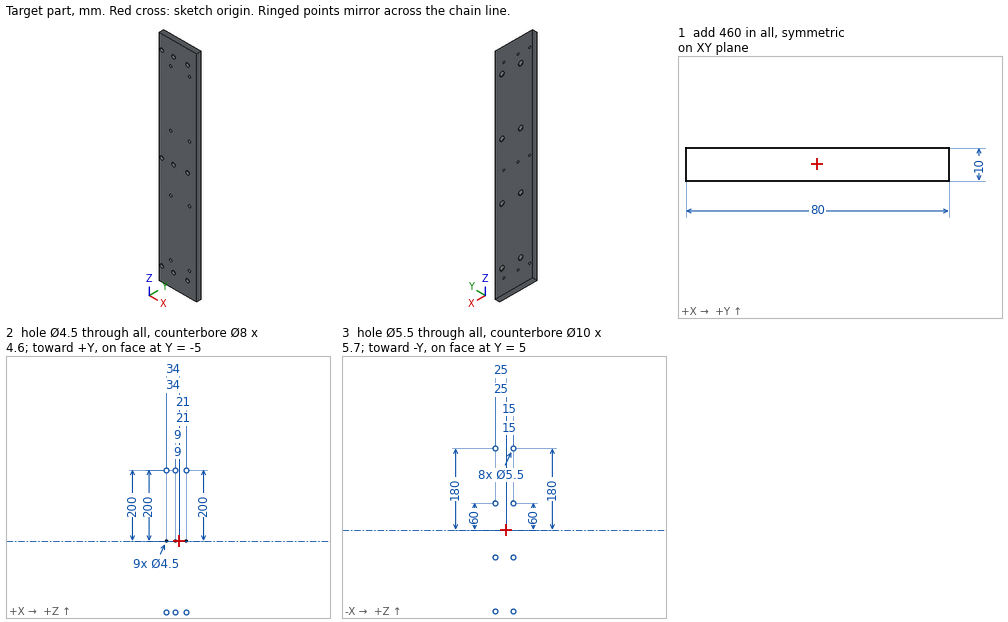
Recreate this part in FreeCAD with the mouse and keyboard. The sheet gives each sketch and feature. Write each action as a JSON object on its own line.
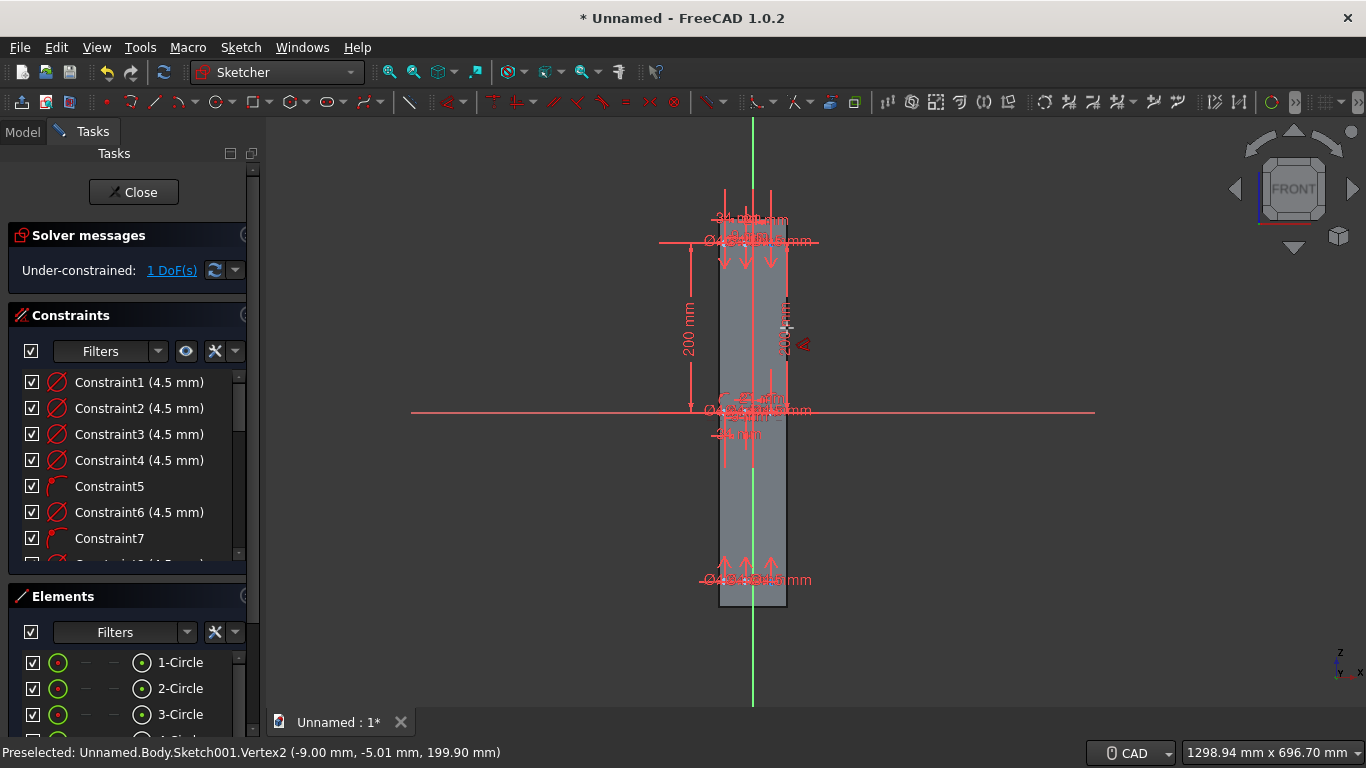
{"action": "left_click", "coordinate": [771, 243]}
{"action": "left_click", "coordinate": [805, 289]}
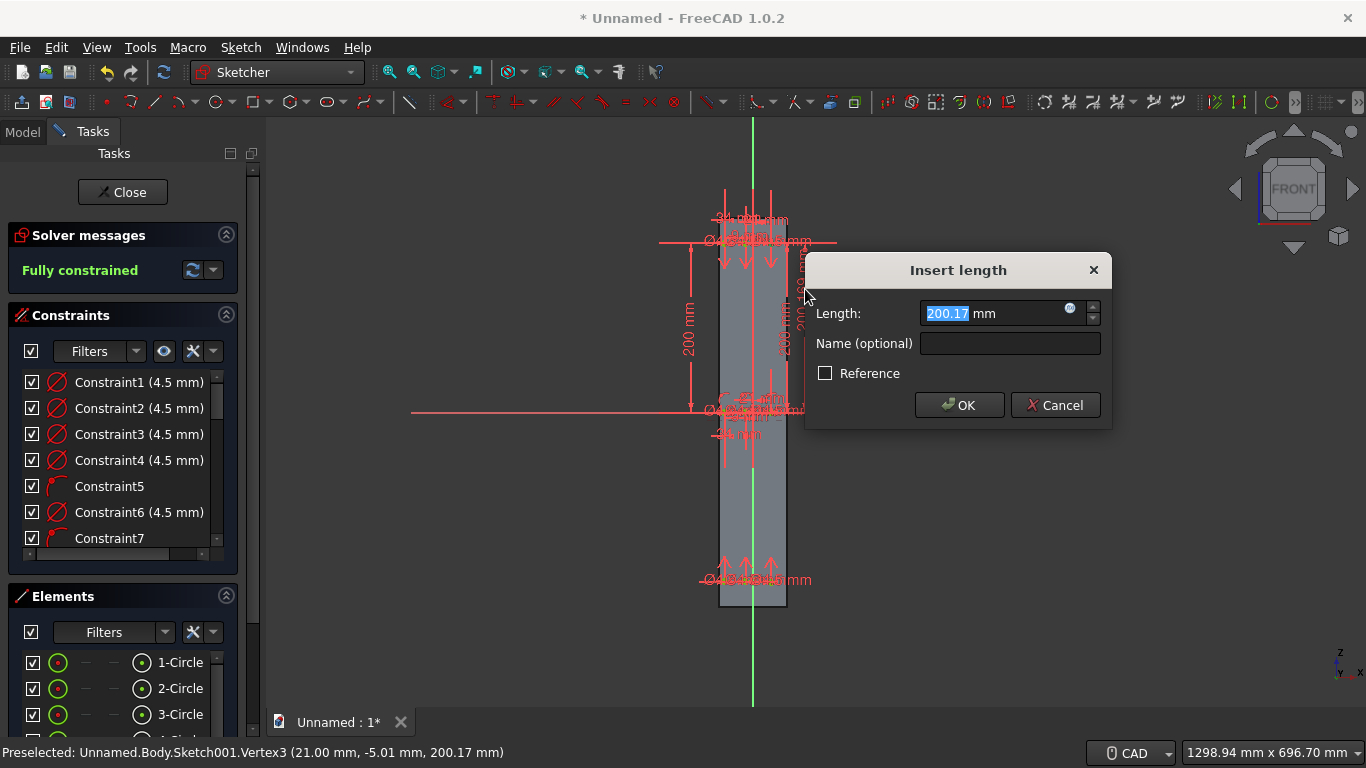
{"action": "type", "text": "200"}
{"action": "key", "text": "Return"}
{"action": "key", "text": "Escape"}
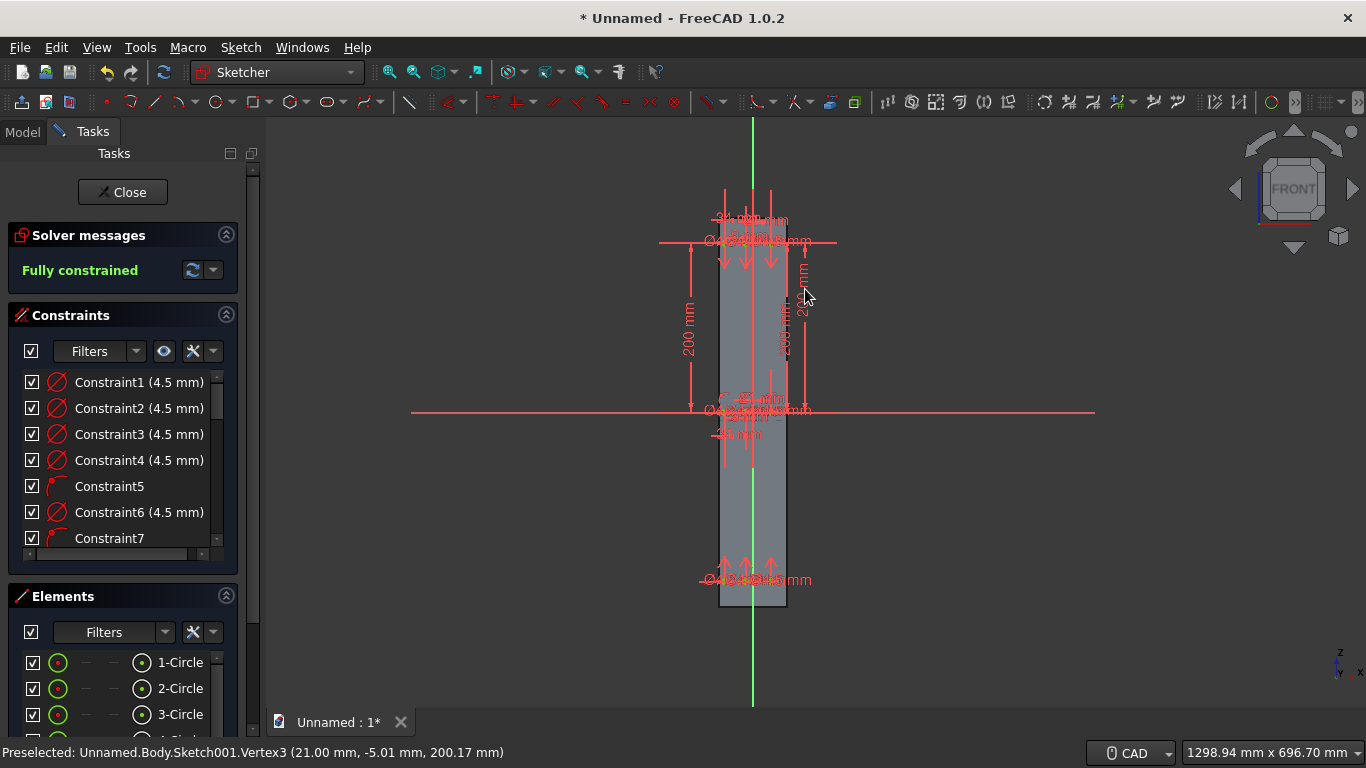
{"action": "left_click", "coordinate": [123, 192]}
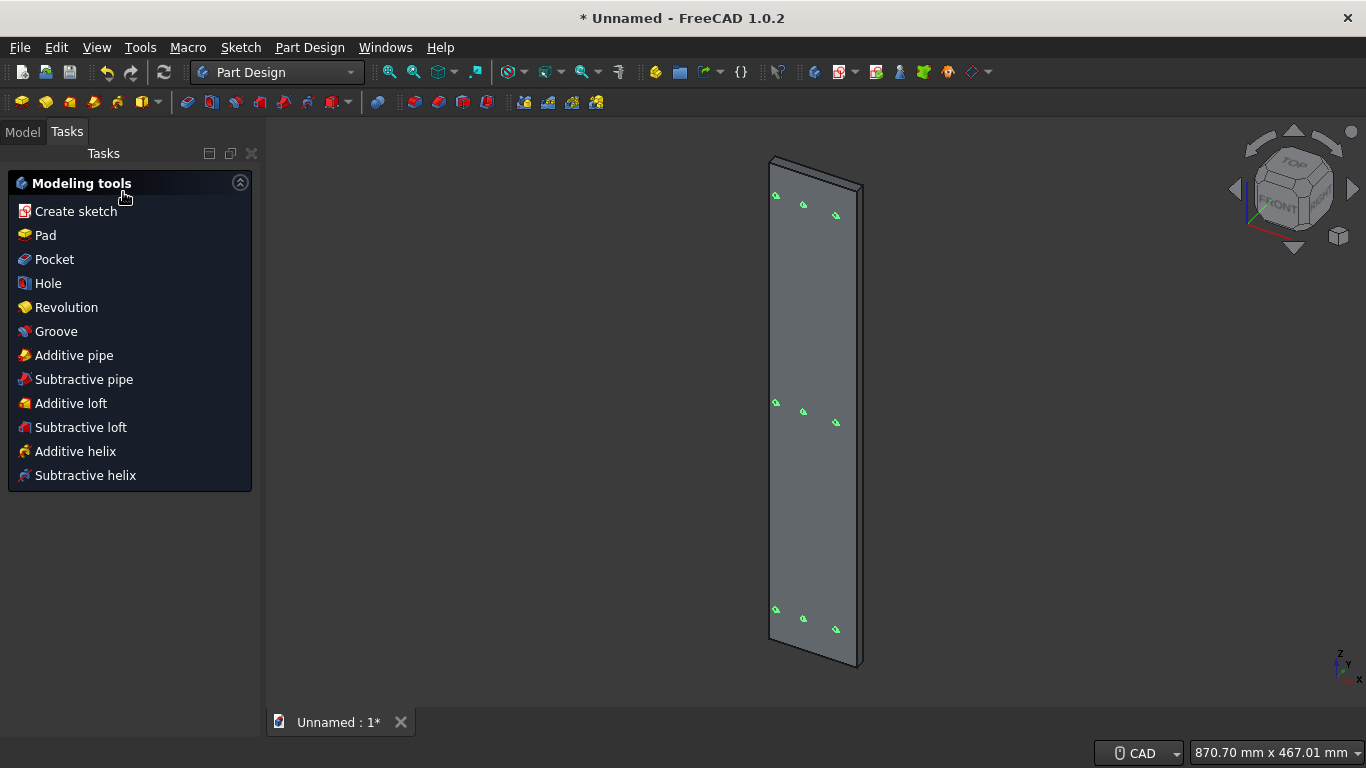
{"action": "left_click", "coordinate": [212, 102]}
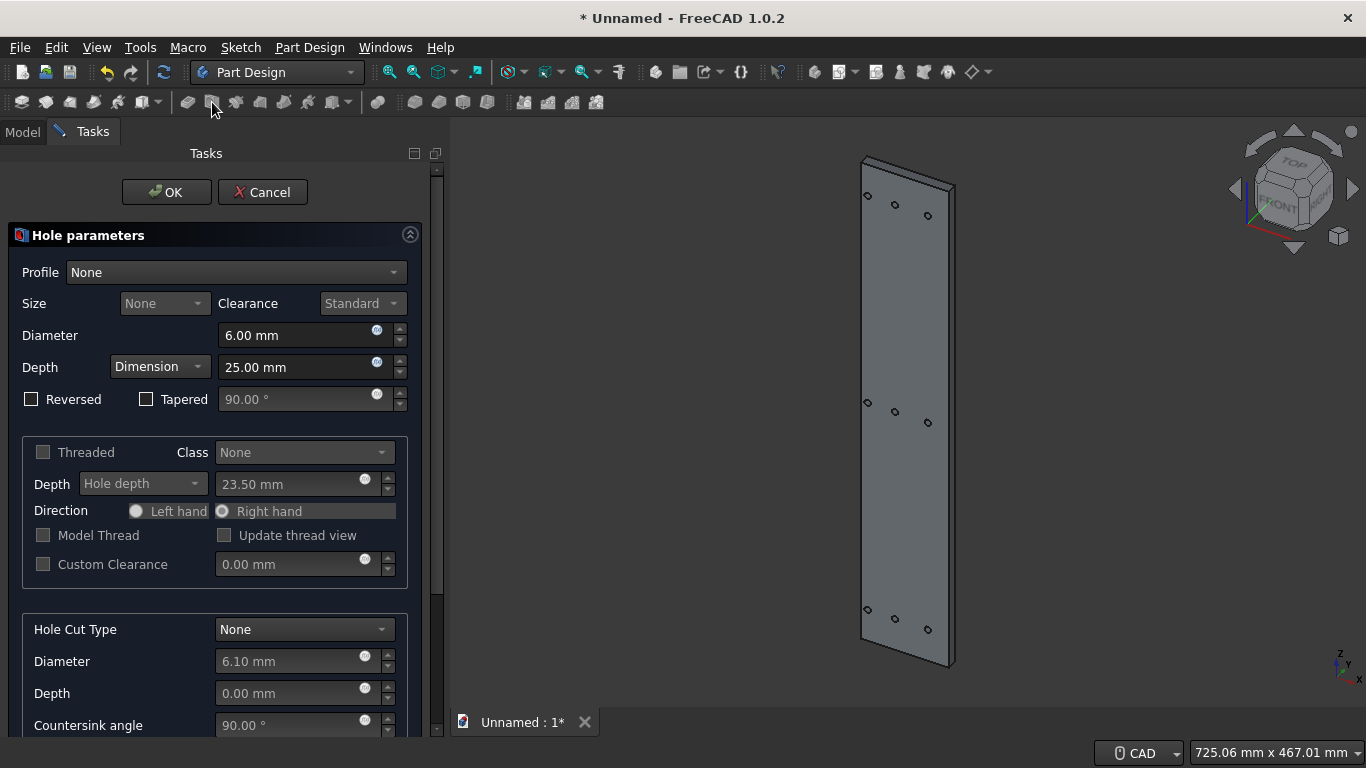
{"action": "triple_click", "coordinate": [305, 335]}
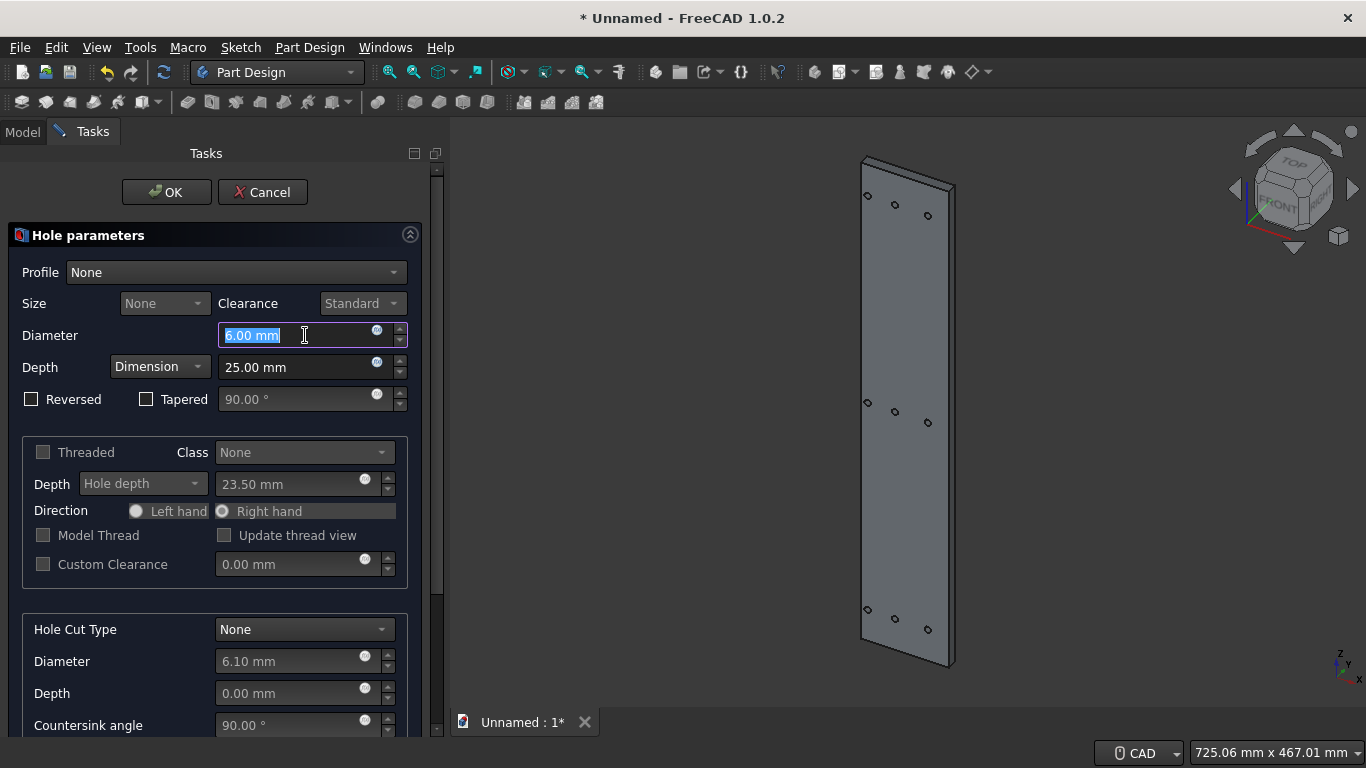
{"action": "type", "text": "4.5"}
{"action": "key", "text": "Tab"}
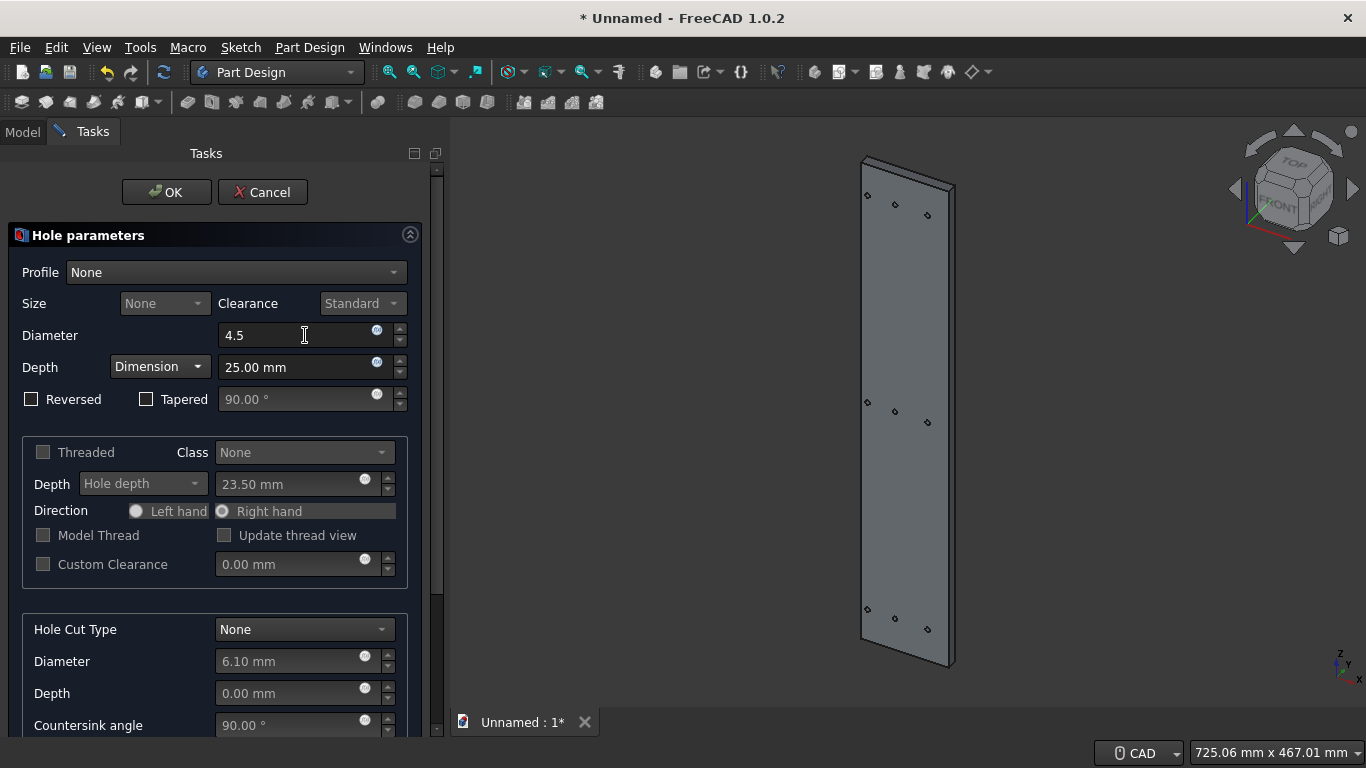
{"action": "left_click", "coordinate": [161, 366]}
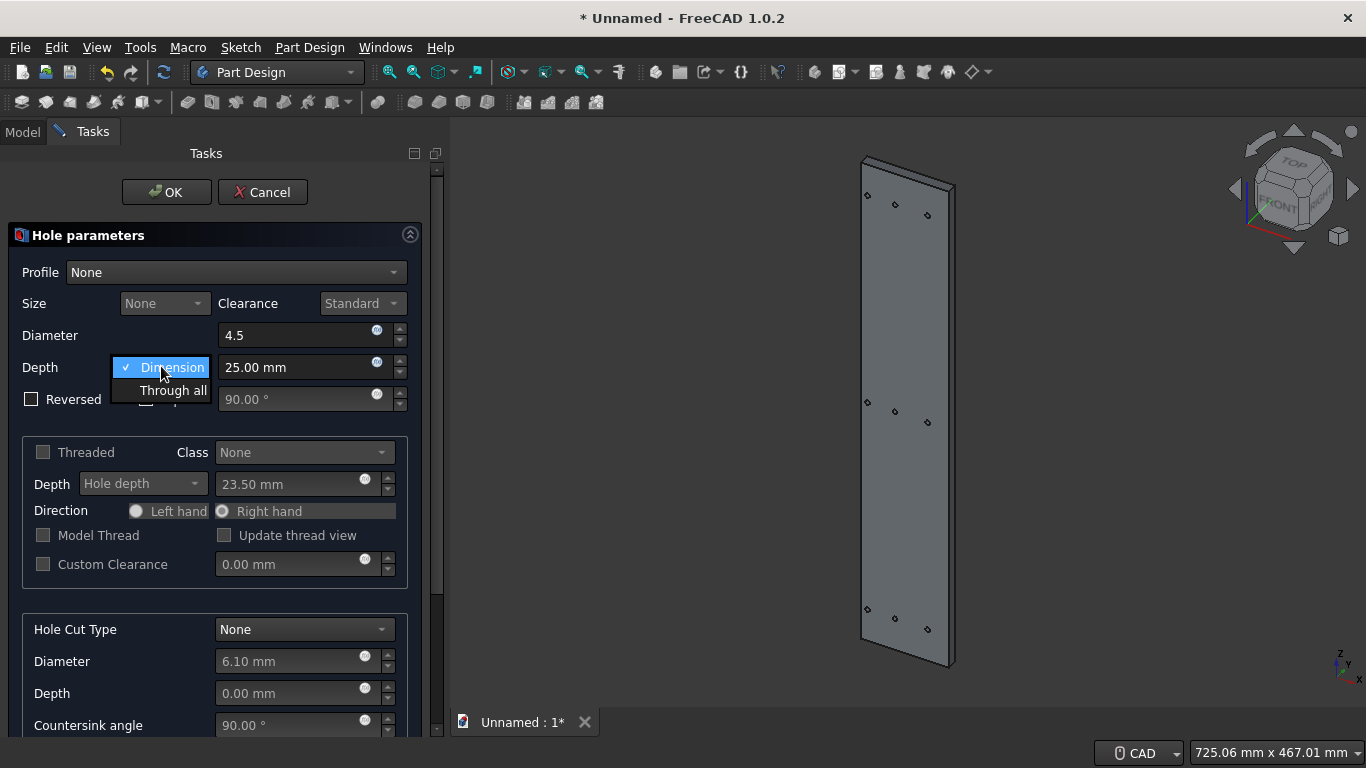
{"action": "left_click", "coordinate": [160, 390]}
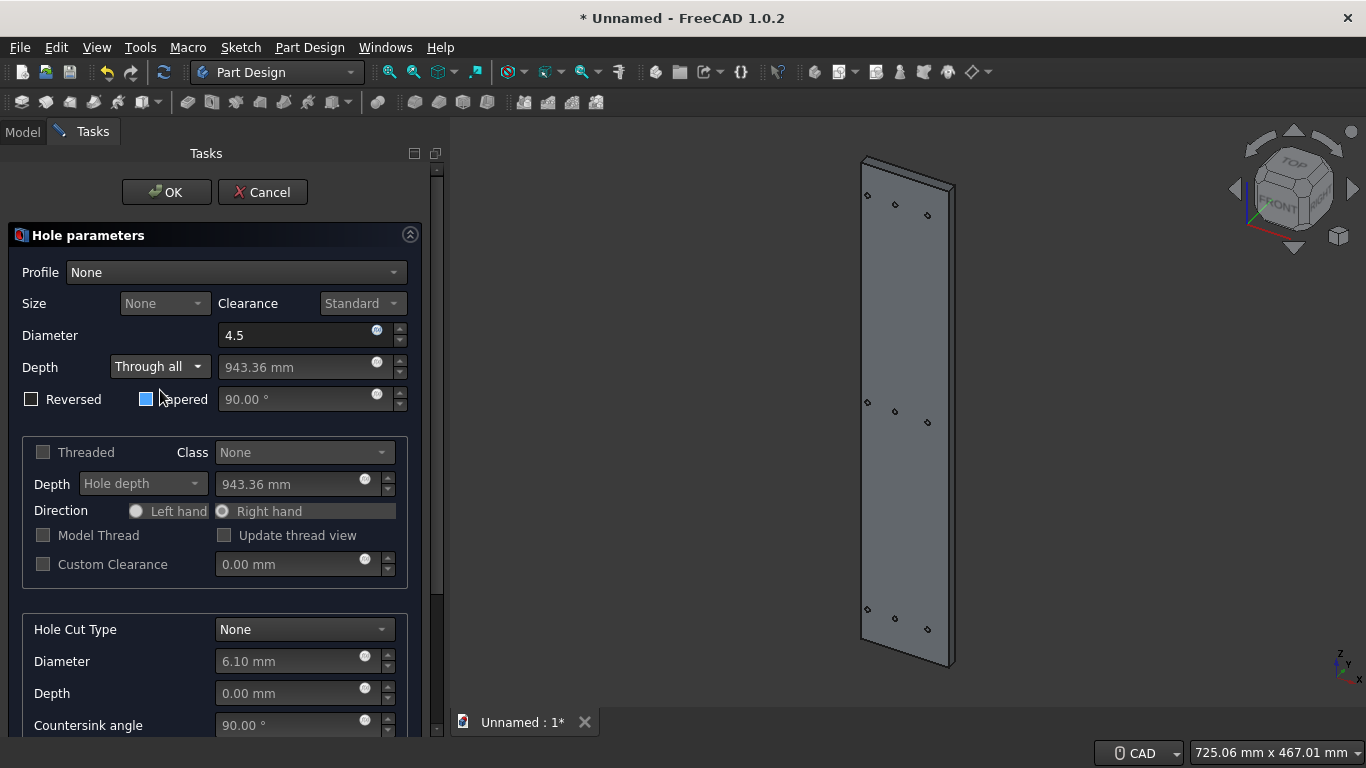
{"action": "left_click", "coordinate": [306, 630]}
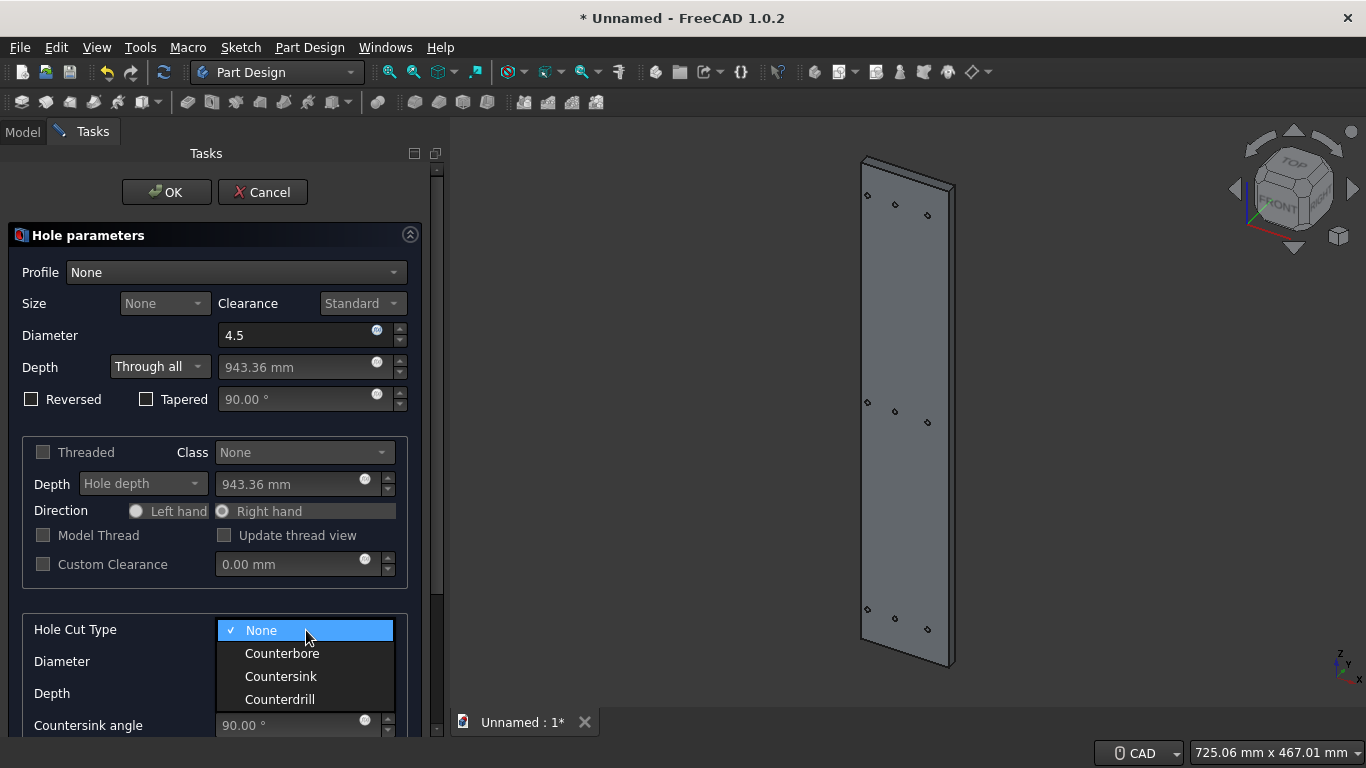
{"action": "left_click", "coordinate": [304, 654]}